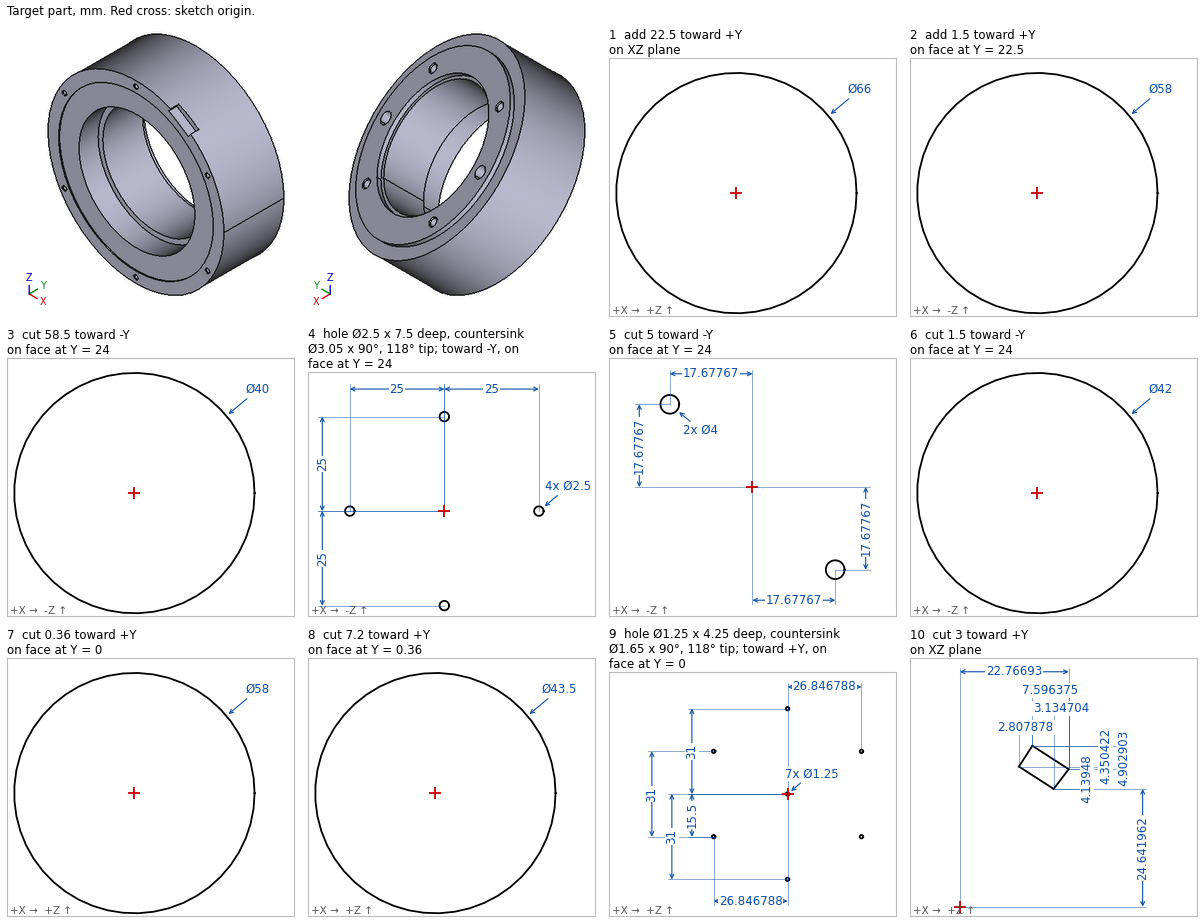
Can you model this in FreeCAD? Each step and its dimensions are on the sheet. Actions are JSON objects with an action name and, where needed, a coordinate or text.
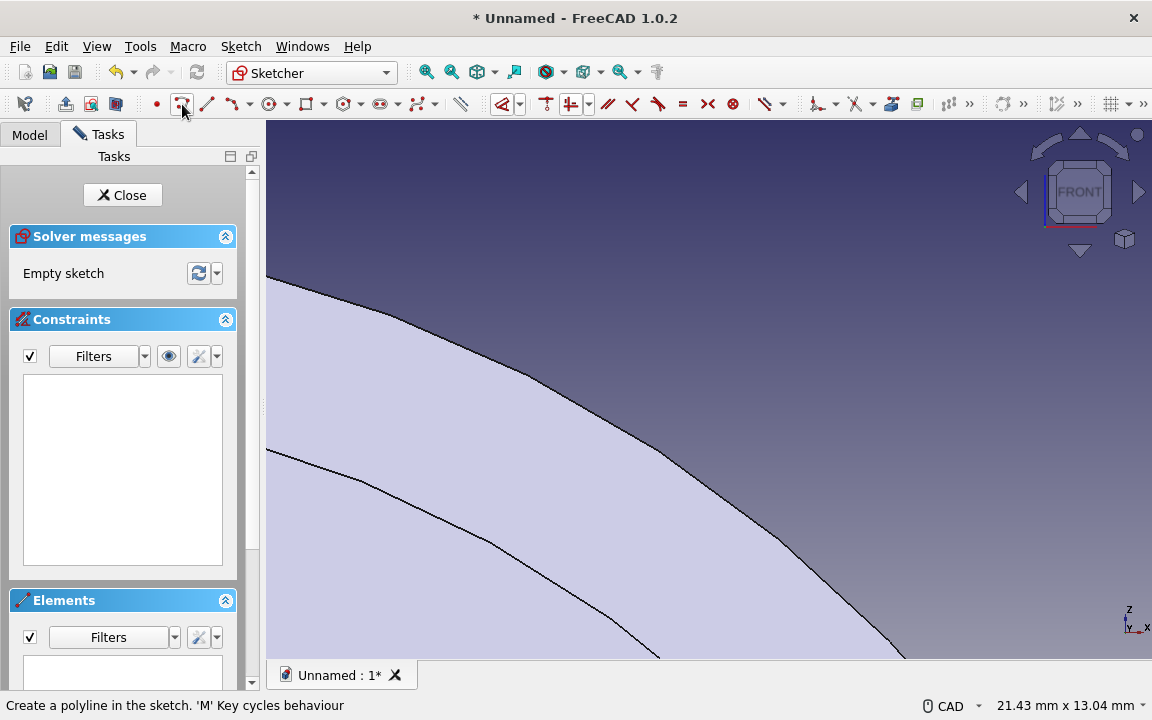
{"action": "left_click", "coordinate": [723, 574]}
{"action": "left_click", "coordinate": [853, 403]}
{"action": "left_click", "coordinate": [539, 200]}
{"action": "left_click", "coordinate": [423, 380]}
{"action": "left_click", "coordinate": [723, 575]}
{"action": "key", "text": "Escape"}
{"action": "key", "text": "Escape"}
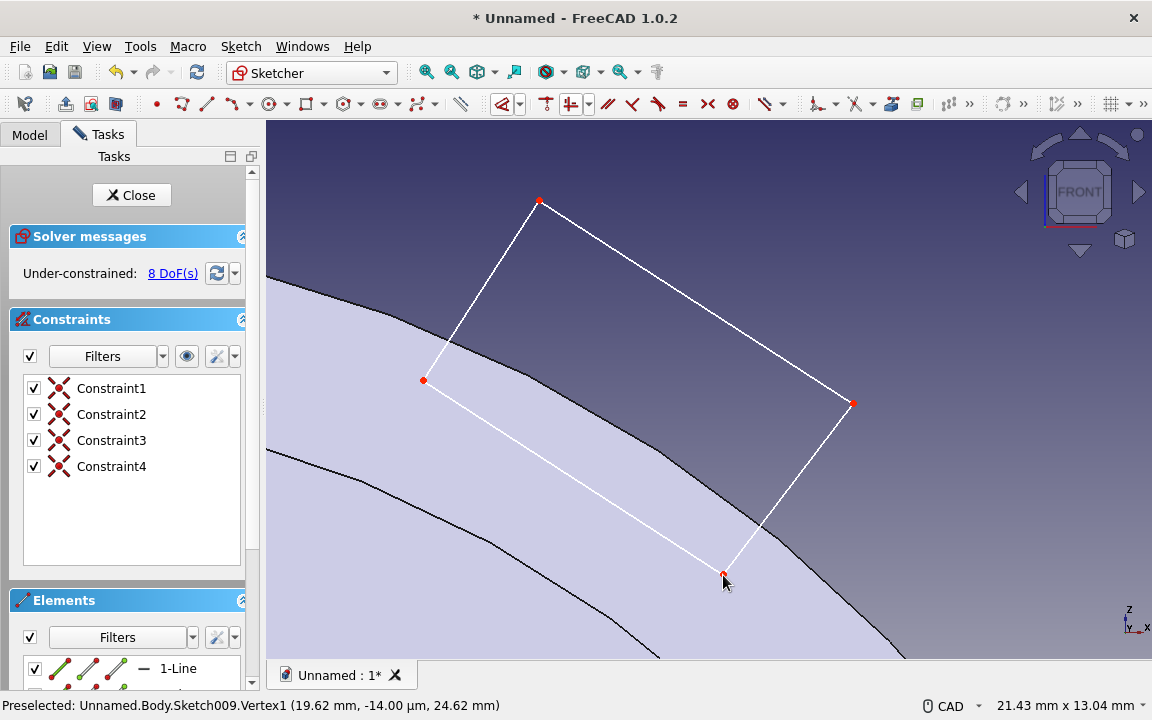
{"action": "left_click", "coordinate": [762, 524]}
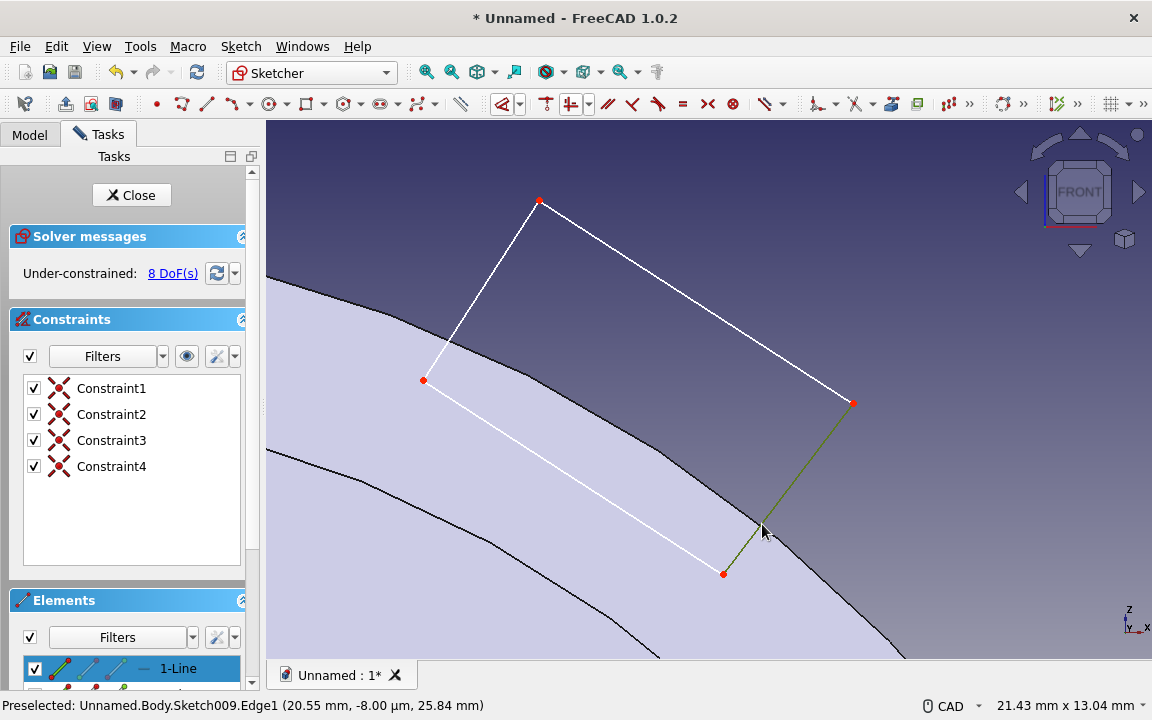
{"action": "key", "text": "i"}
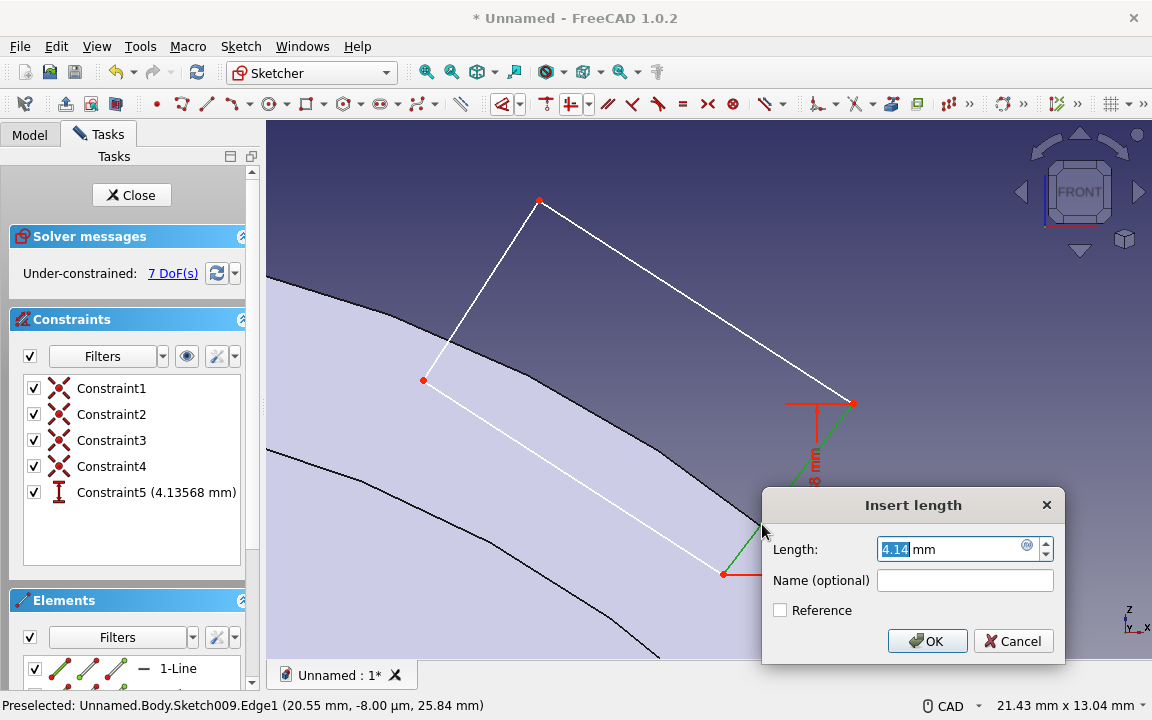
{"action": "type", "text": "4.13948"}
{"action": "key", "text": "Return"}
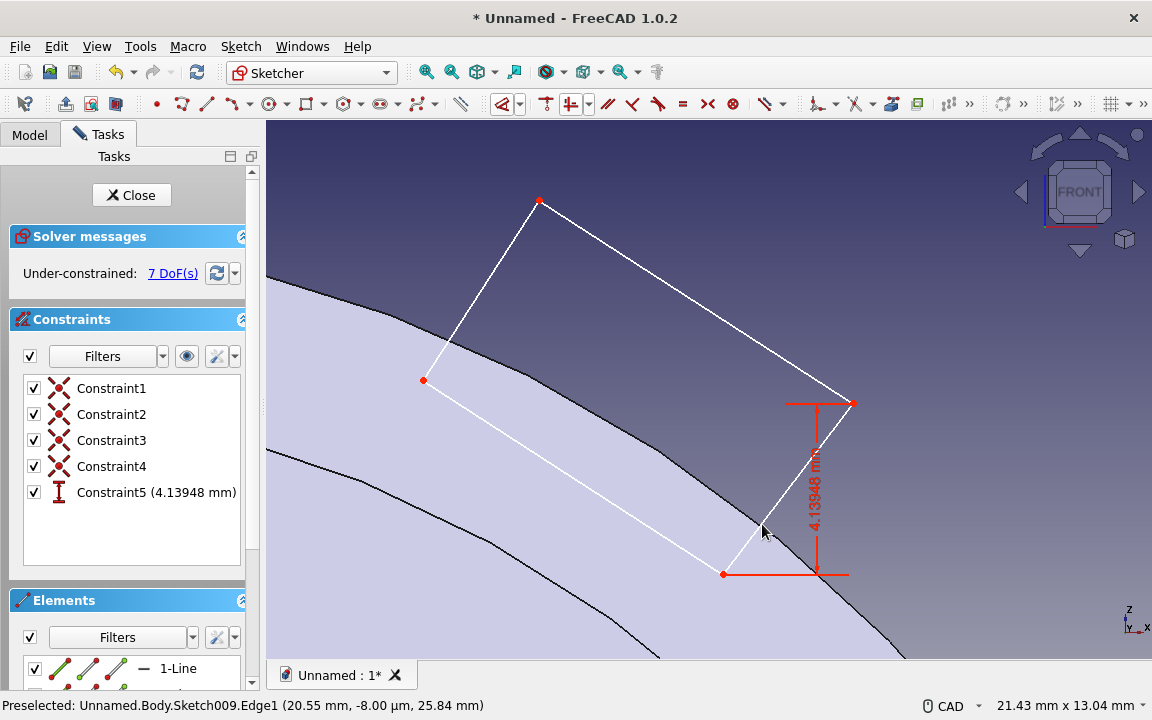
{"action": "left_click", "coordinate": [853, 404]}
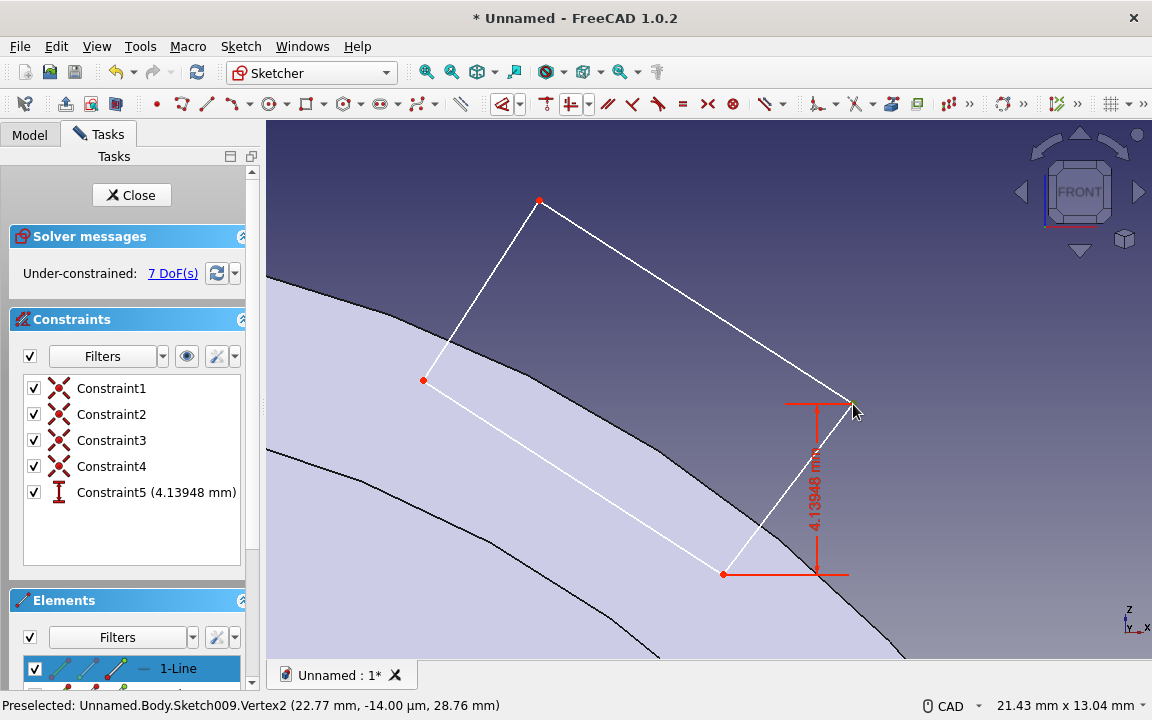
{"action": "key", "text": "l"}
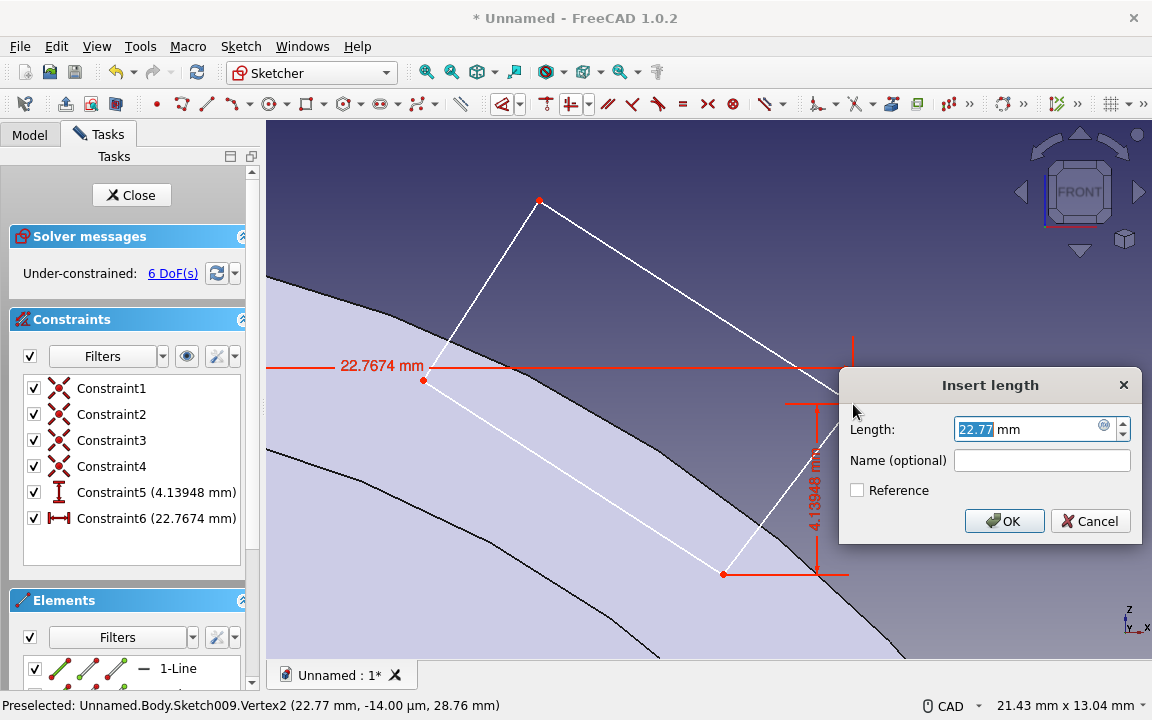
{"action": "type", "text": "22.76693"}
{"action": "key", "text": "Return"}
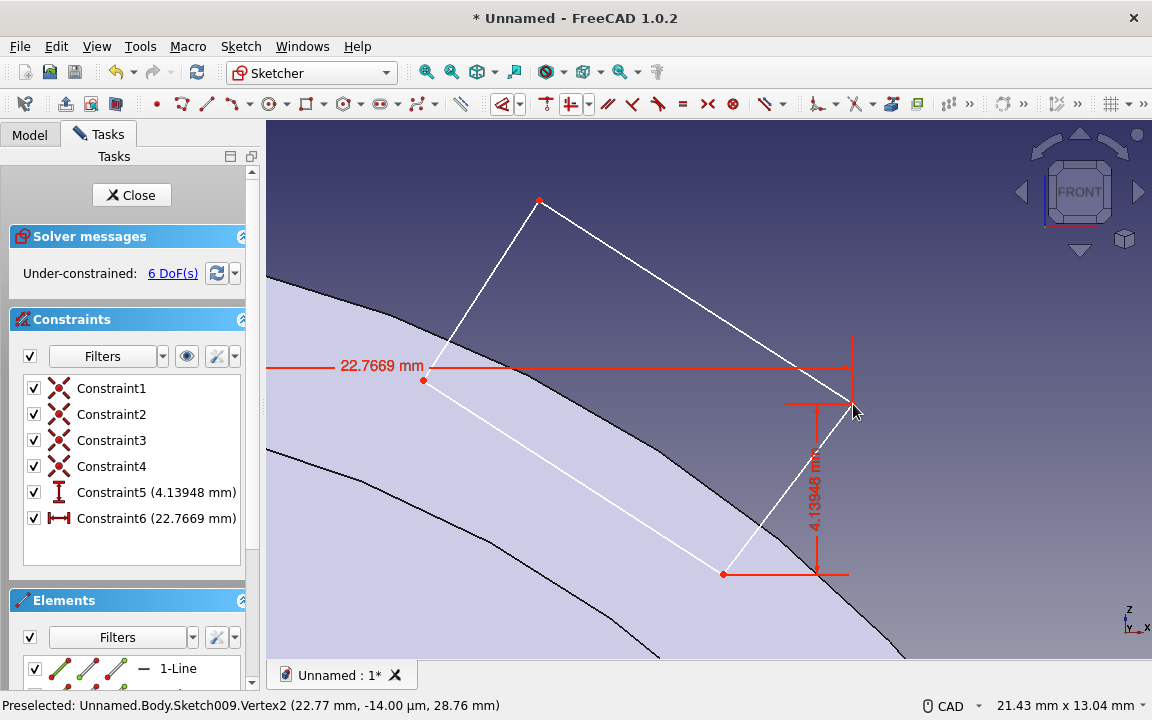
{"action": "left_click", "coordinate": [762, 524]}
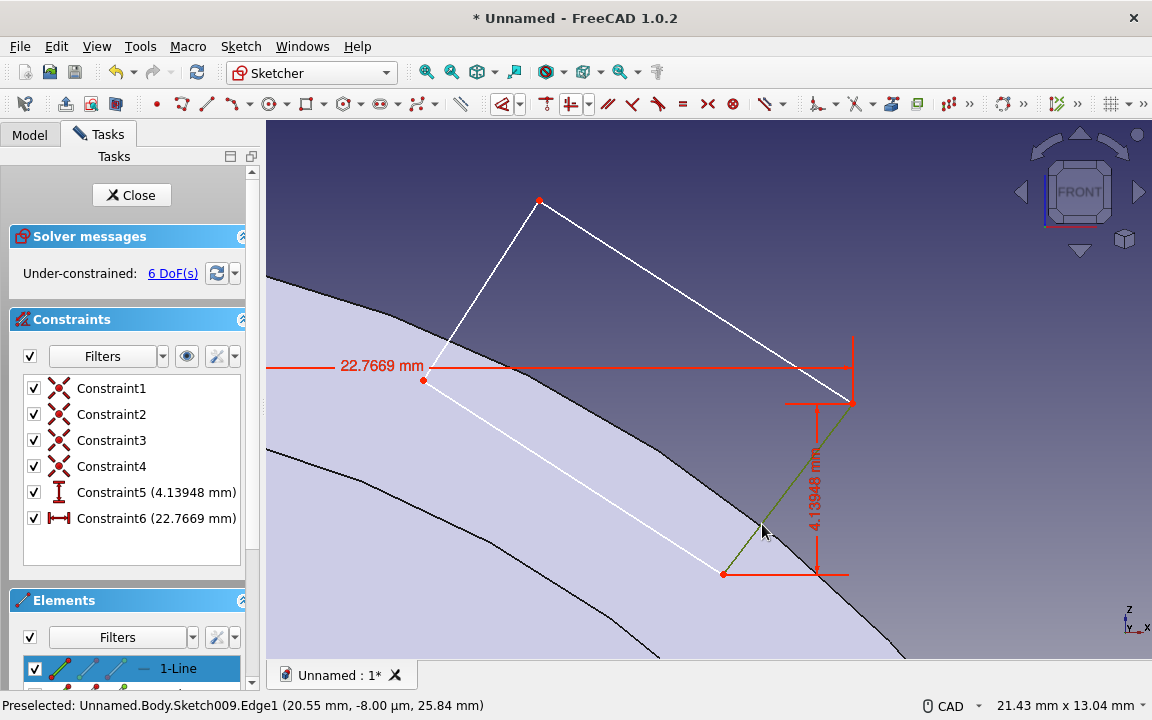
{"action": "left_click", "coordinate": [520, 104]}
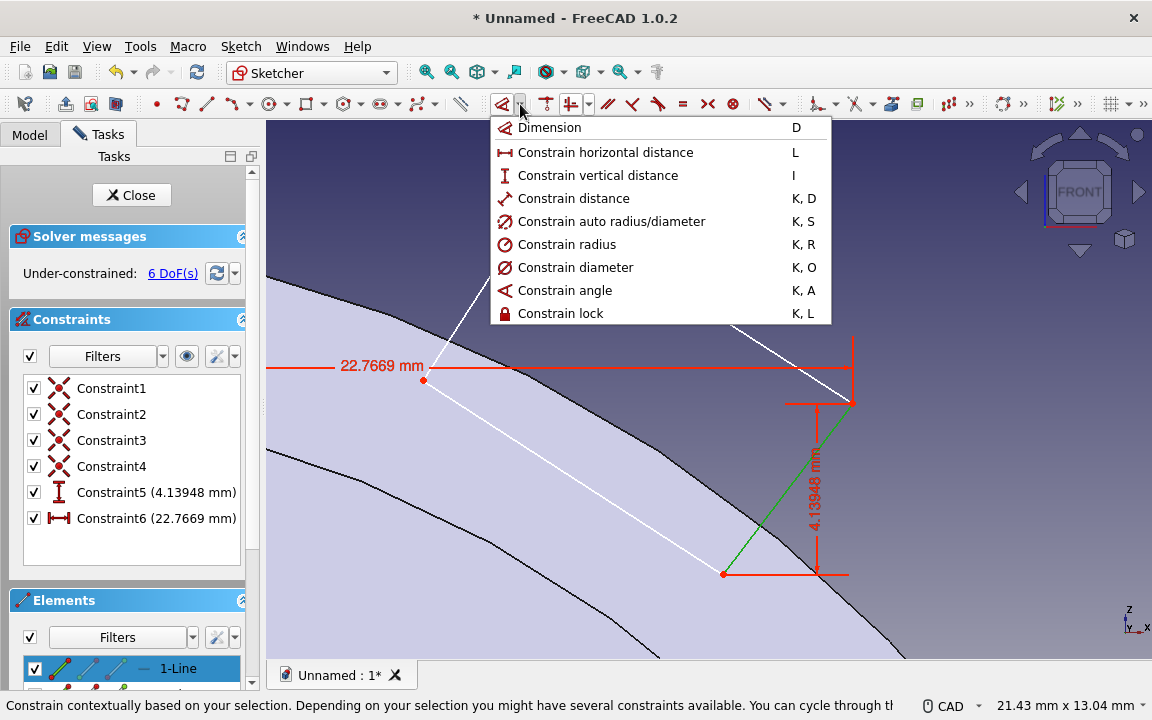
{"action": "left_click", "coordinate": [661, 152]}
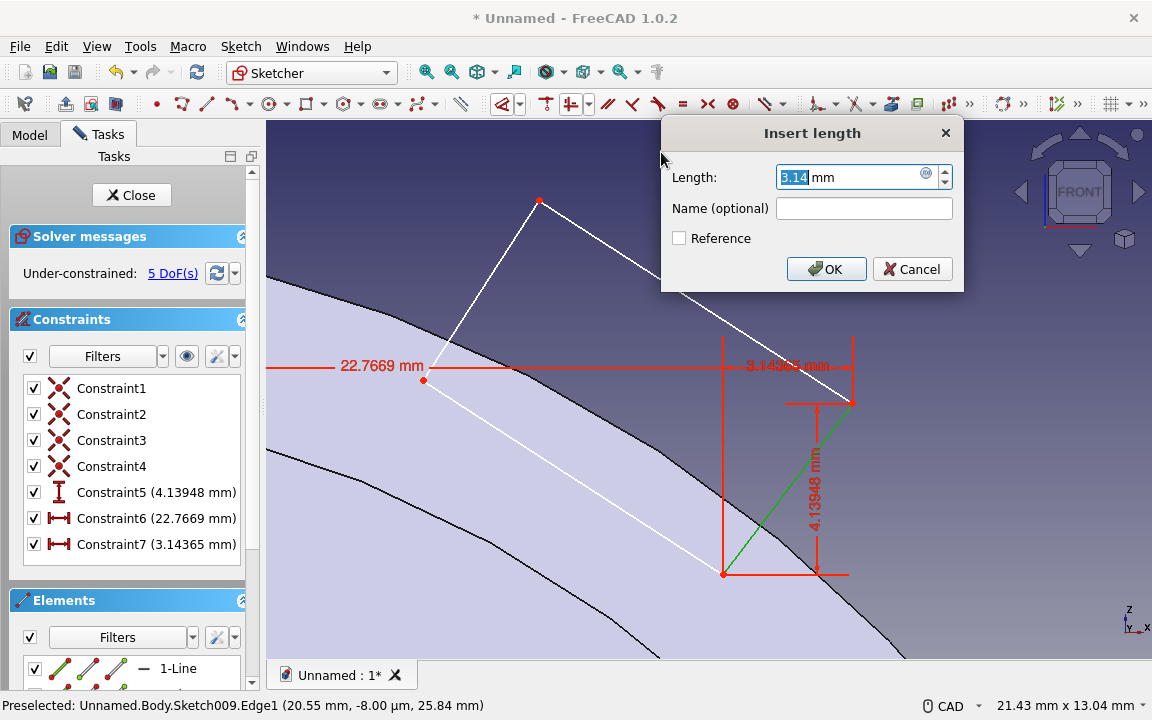
{"action": "type", "text": "3.134704"}
{"action": "key", "text": "Return"}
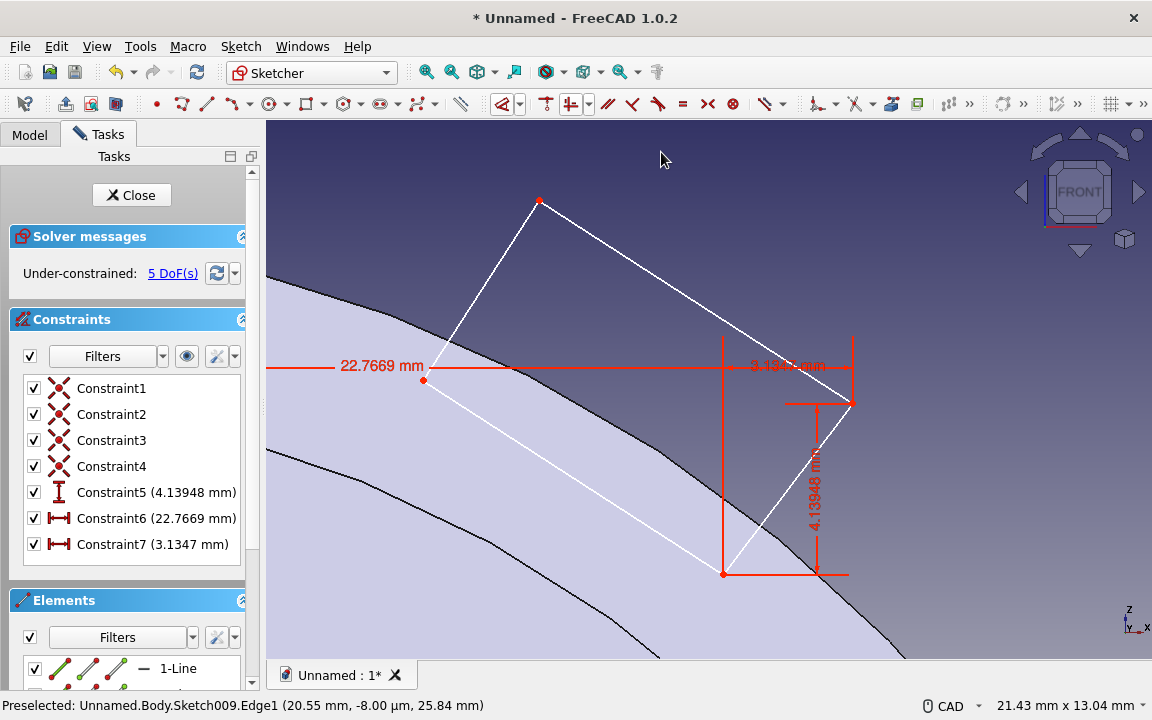
{"action": "left_click", "coordinate": [759, 343]}